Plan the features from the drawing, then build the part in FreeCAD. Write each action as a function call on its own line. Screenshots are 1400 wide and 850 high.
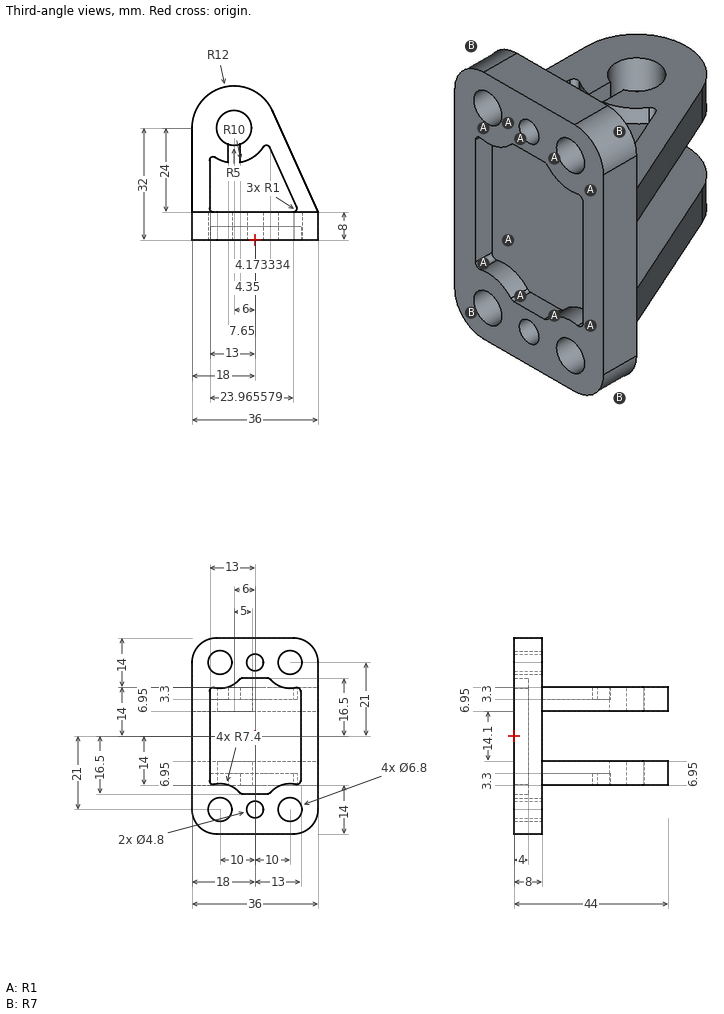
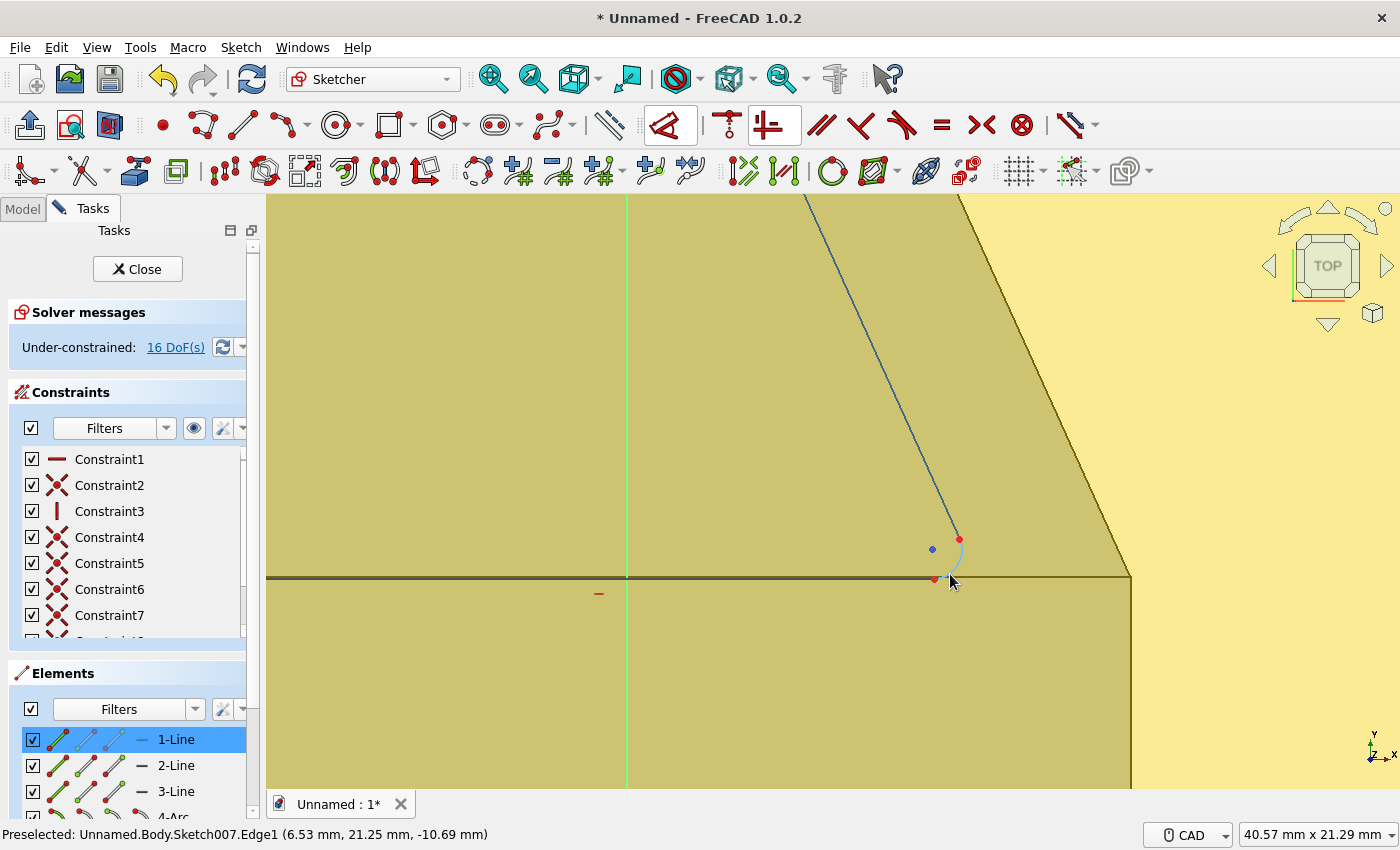
click(950, 573)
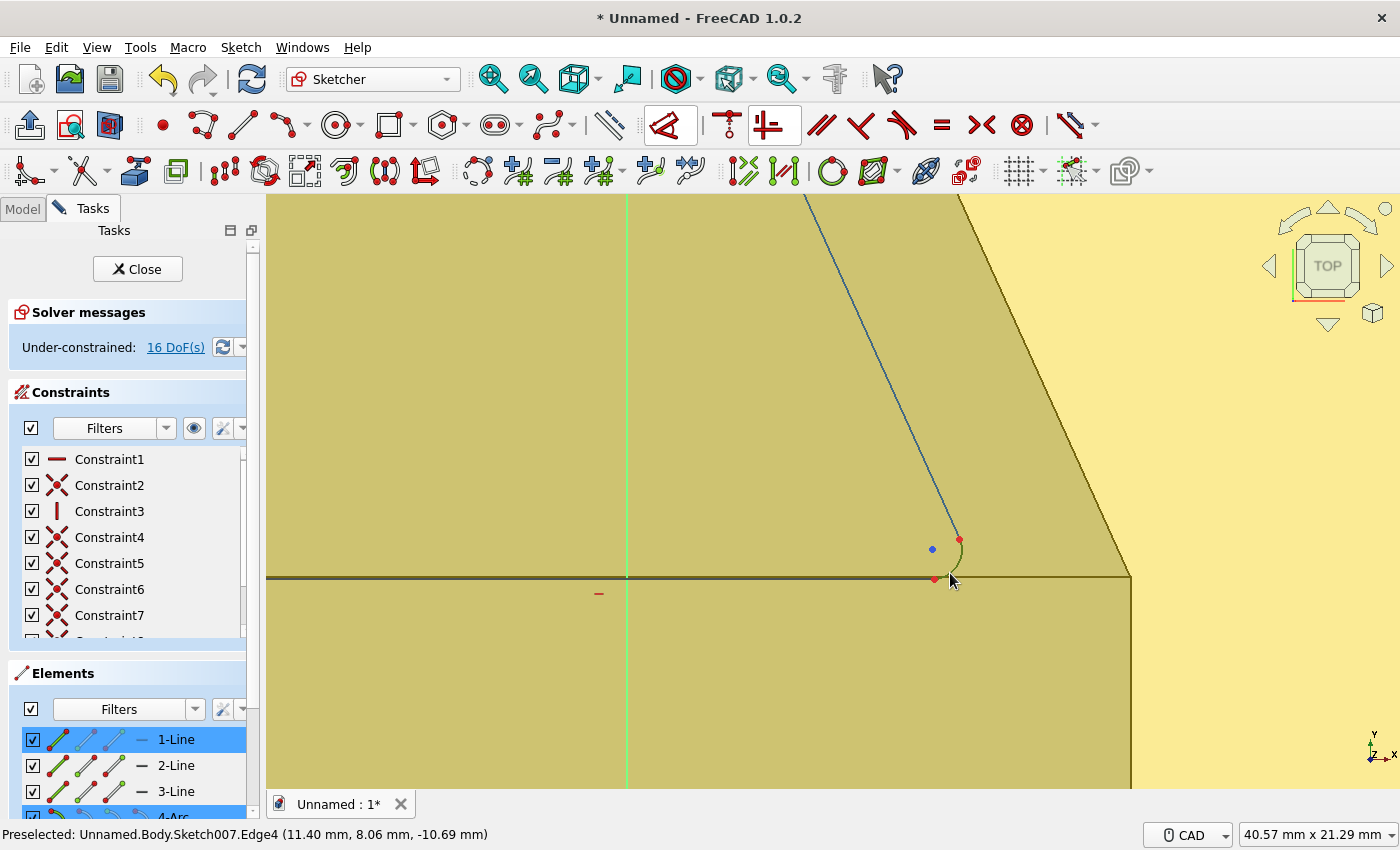
key(t)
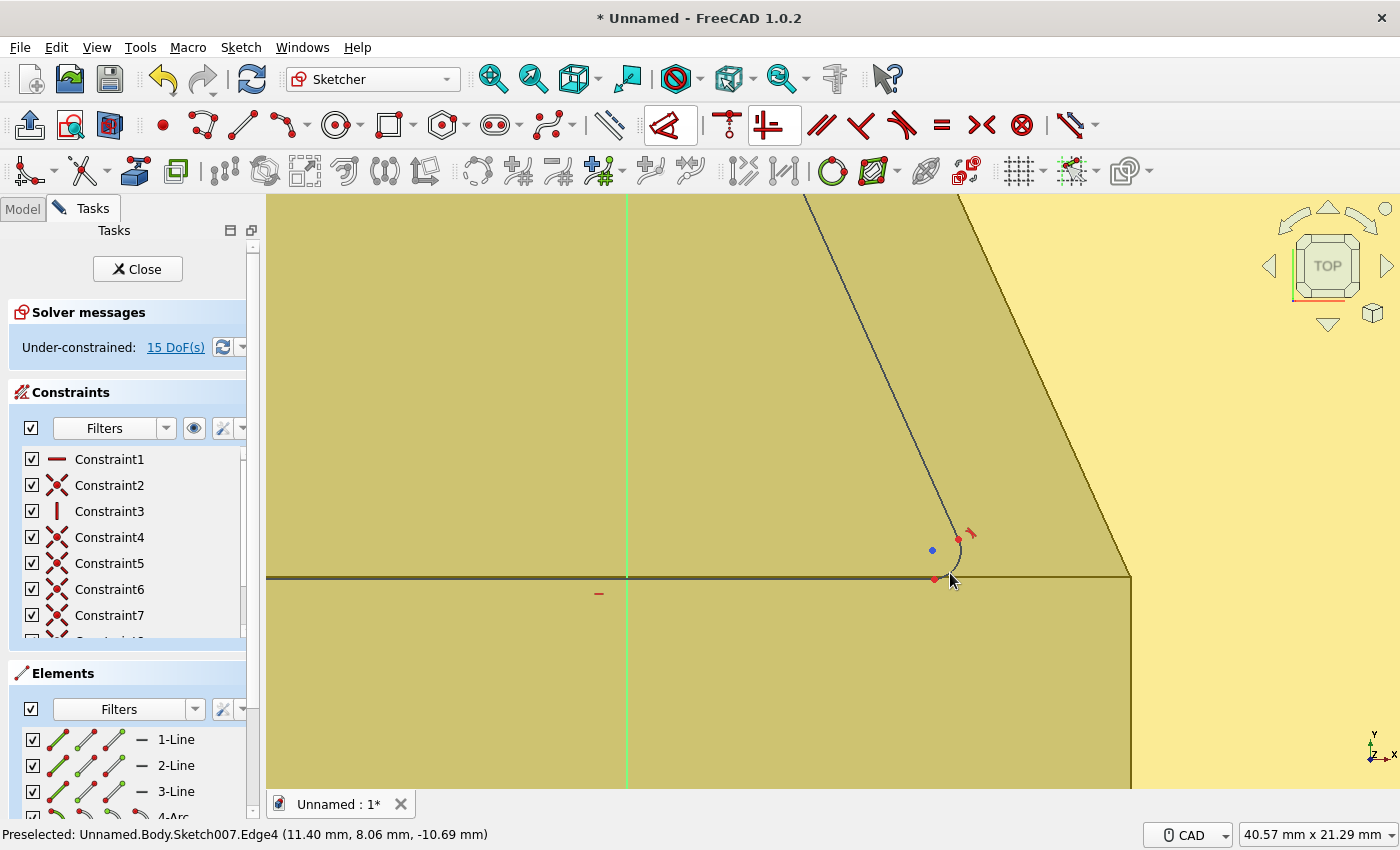
click(894, 396)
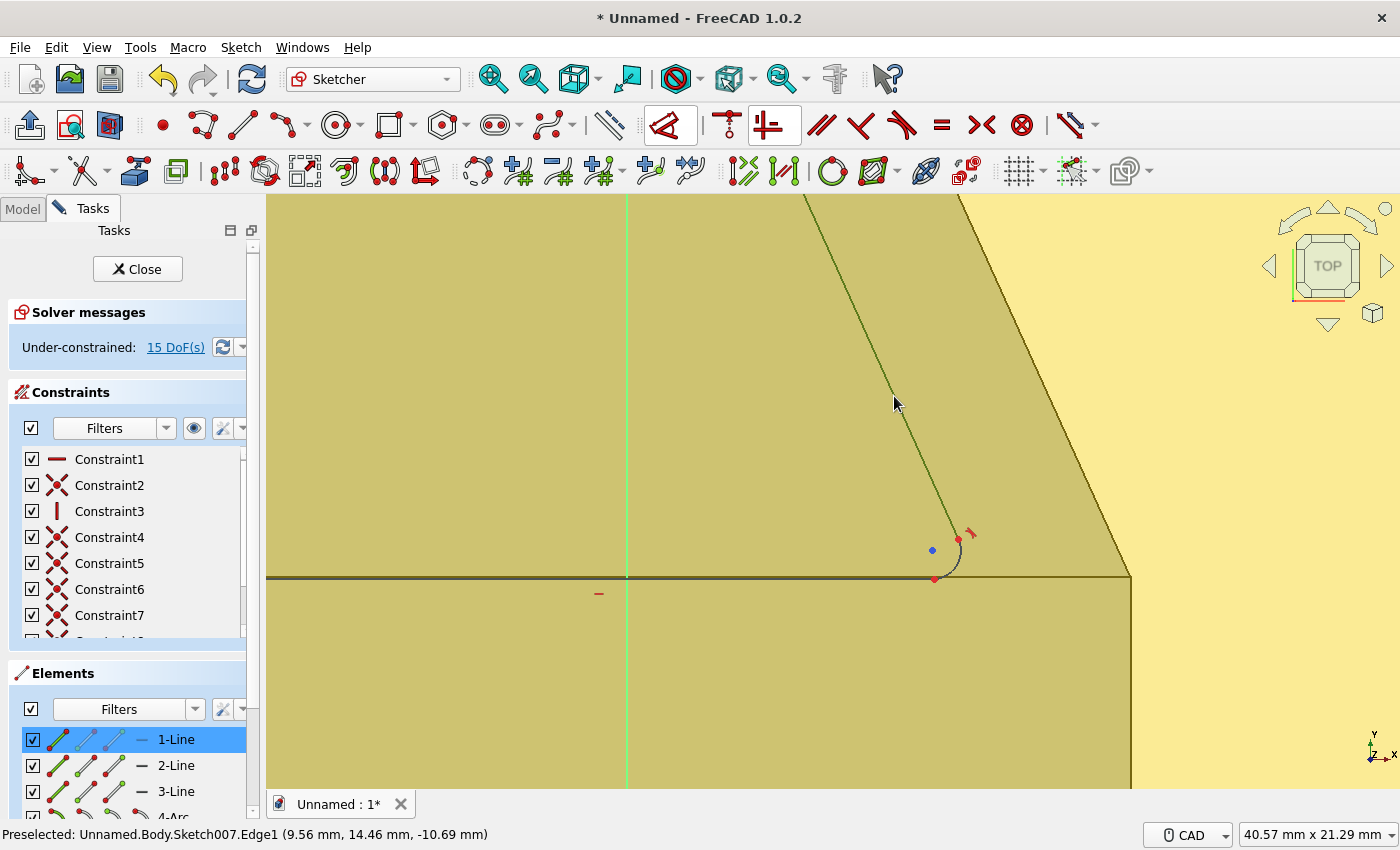
scroll(950, 575, down, 3)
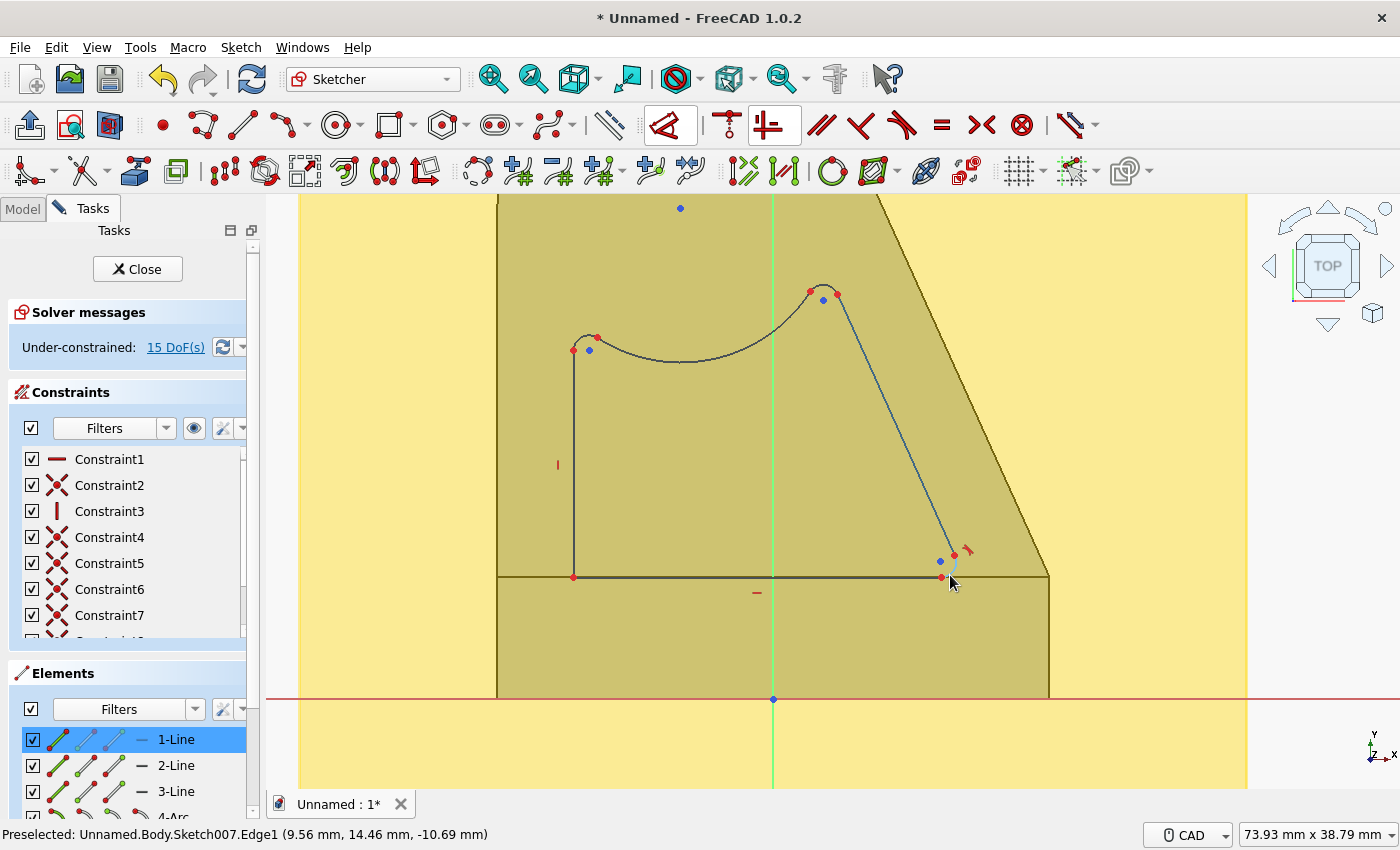
scroll(831, 287, up, 2)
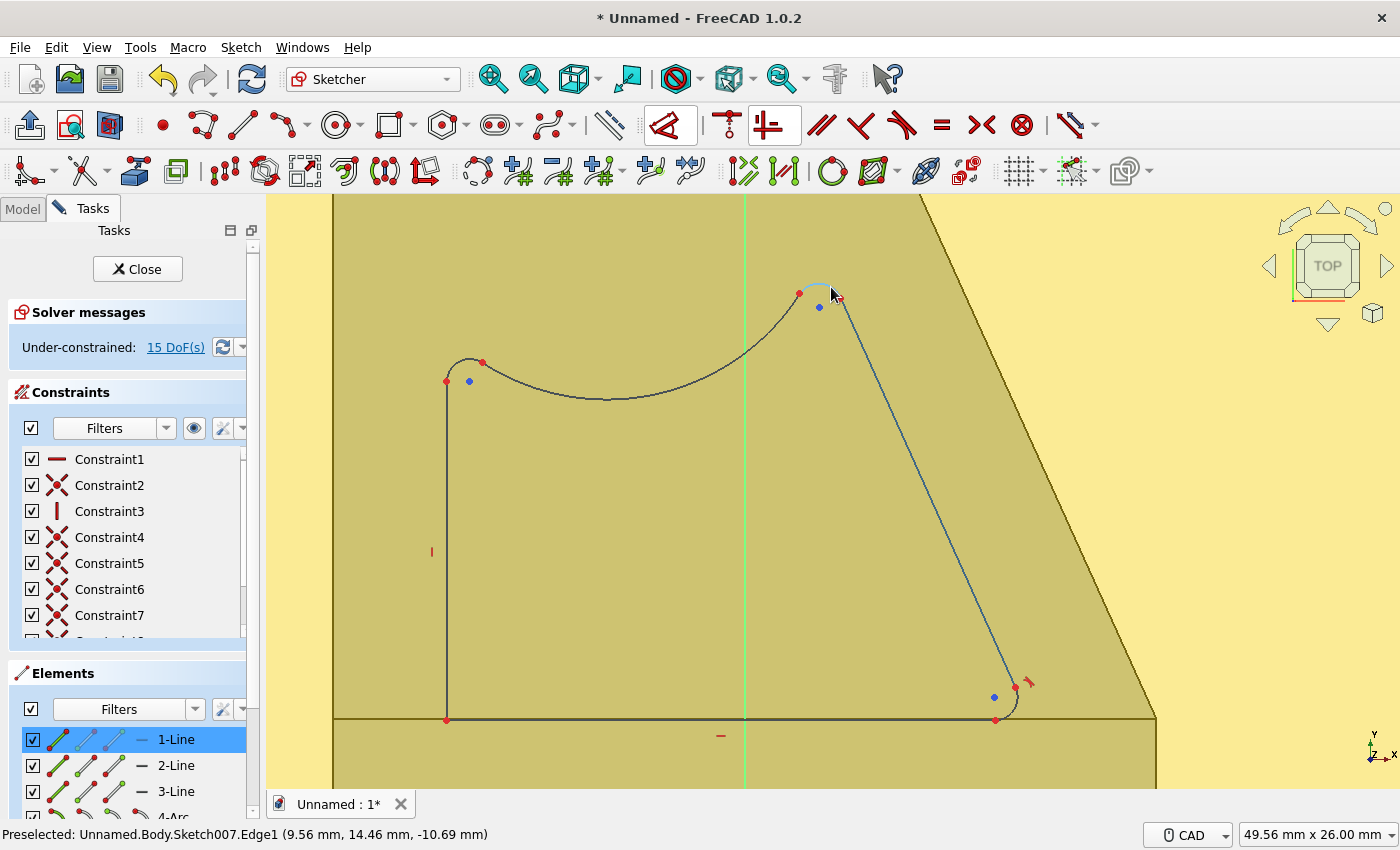
click(831, 287)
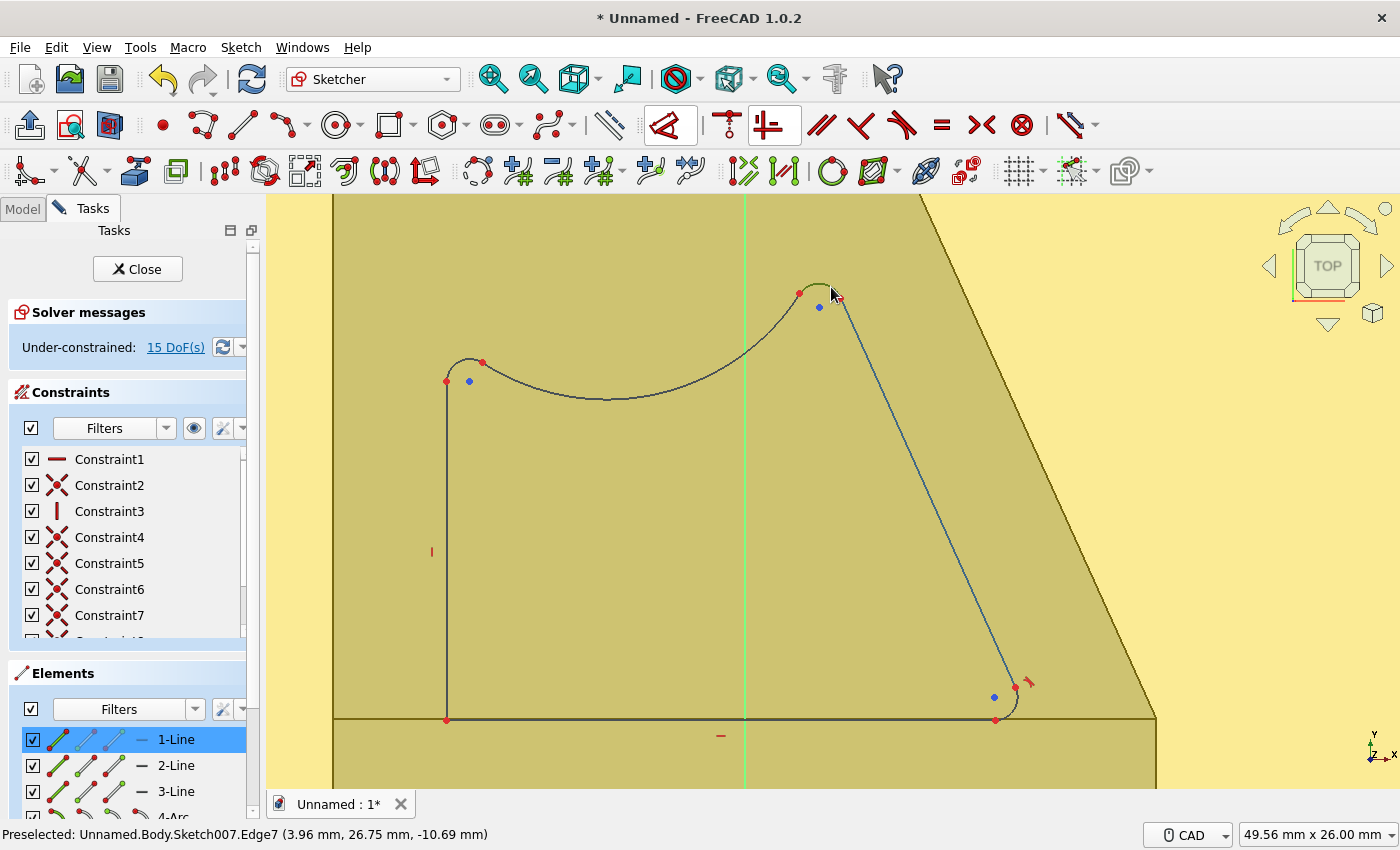
key(t)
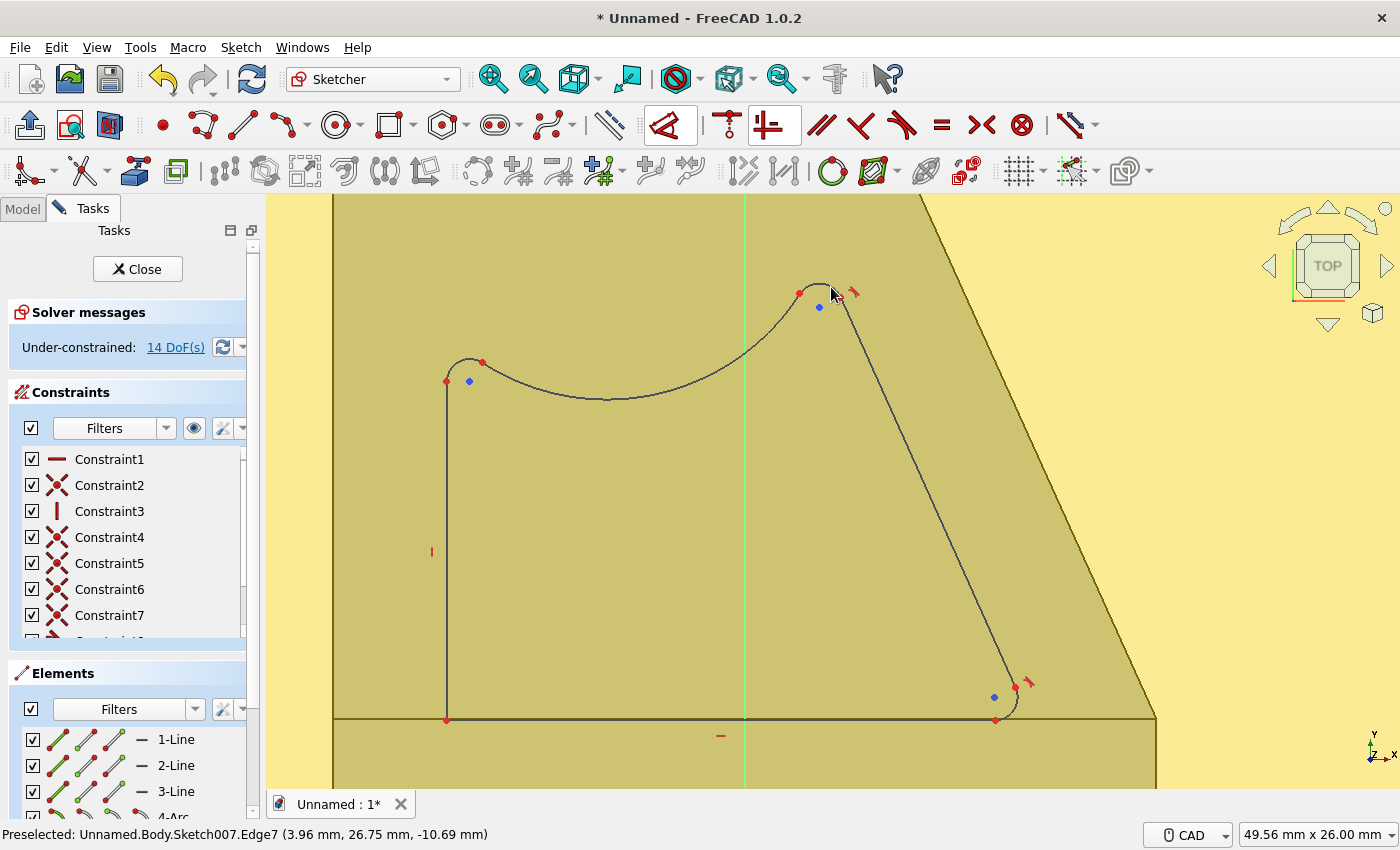
click(831, 720)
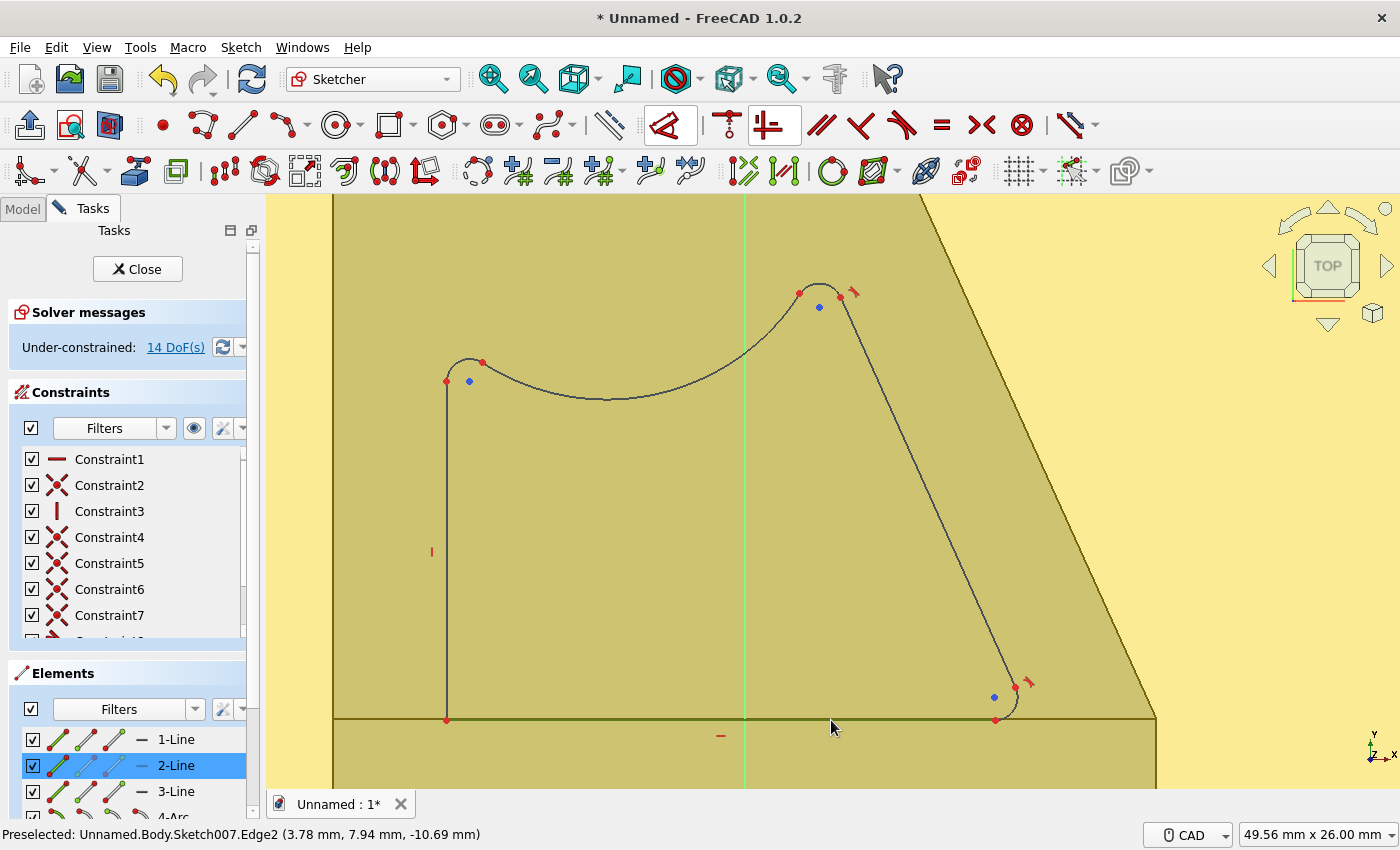
click(1008, 716)